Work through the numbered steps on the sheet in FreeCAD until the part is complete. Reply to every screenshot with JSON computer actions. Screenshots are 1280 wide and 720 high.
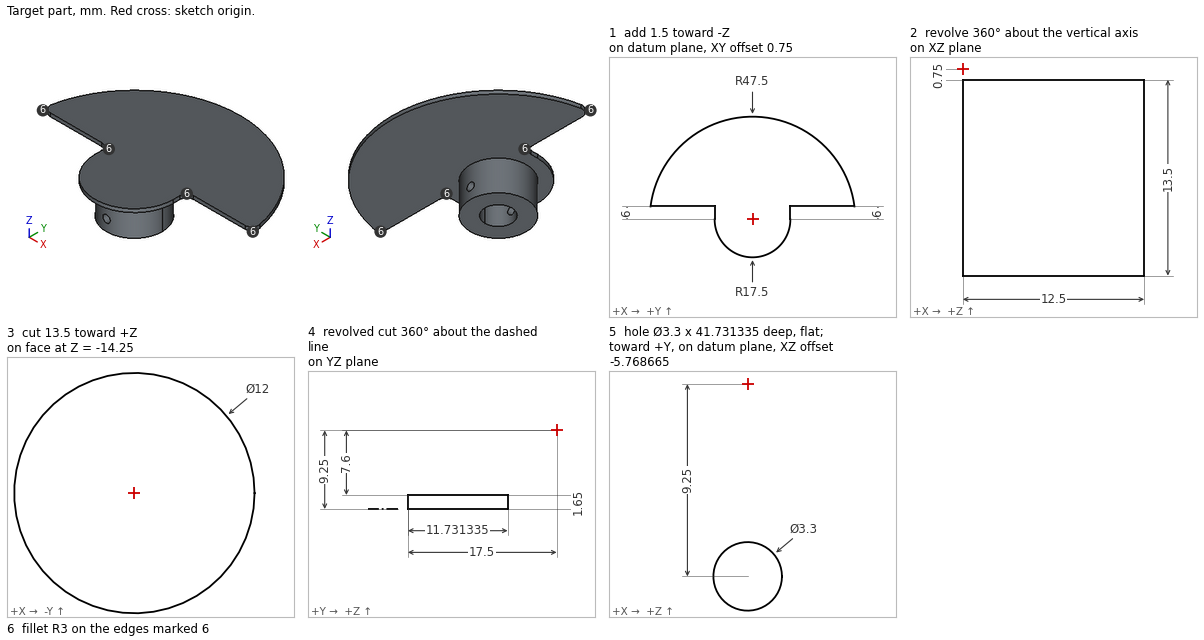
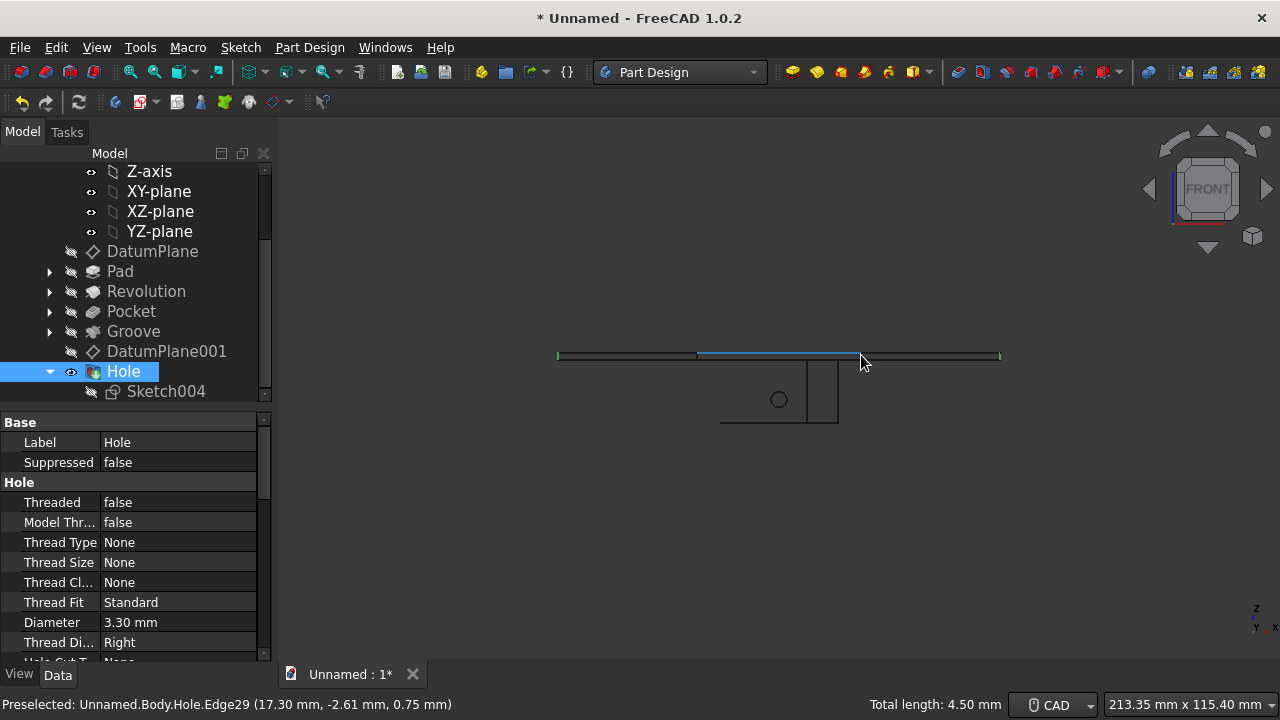
{"action": "key", "text": "3"}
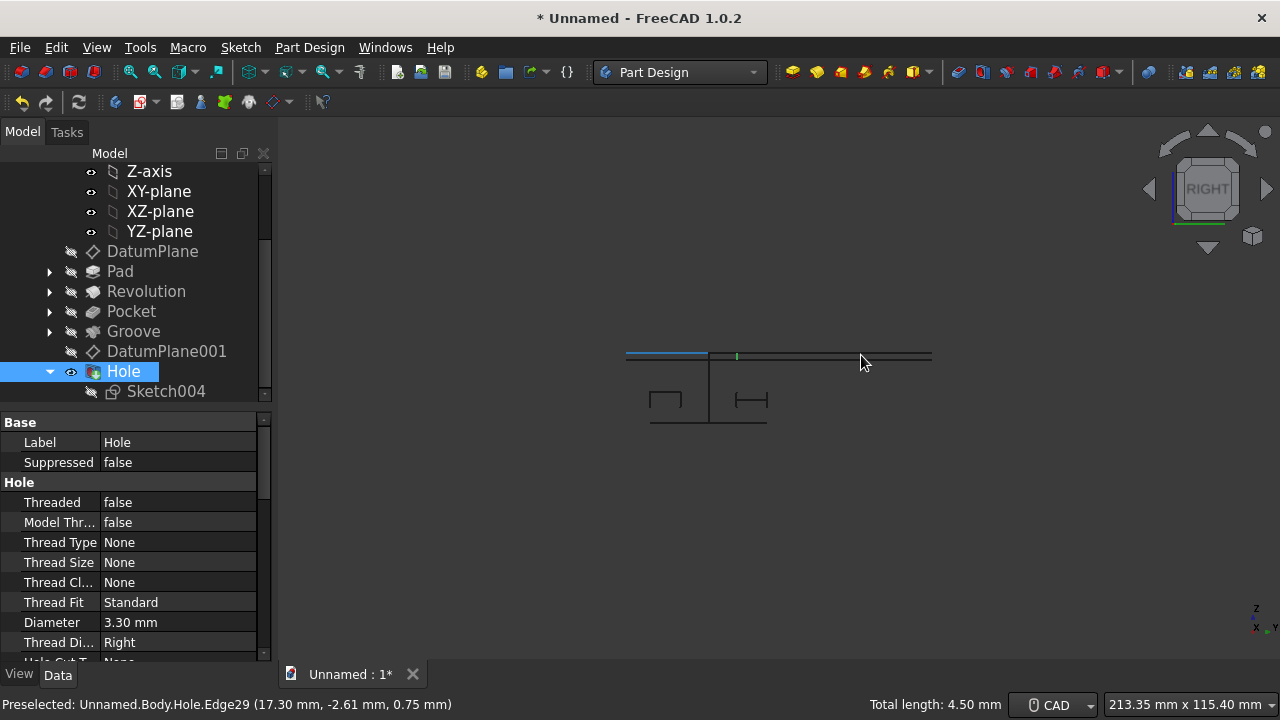
{"action": "left_click", "coordinate": [132, 72]}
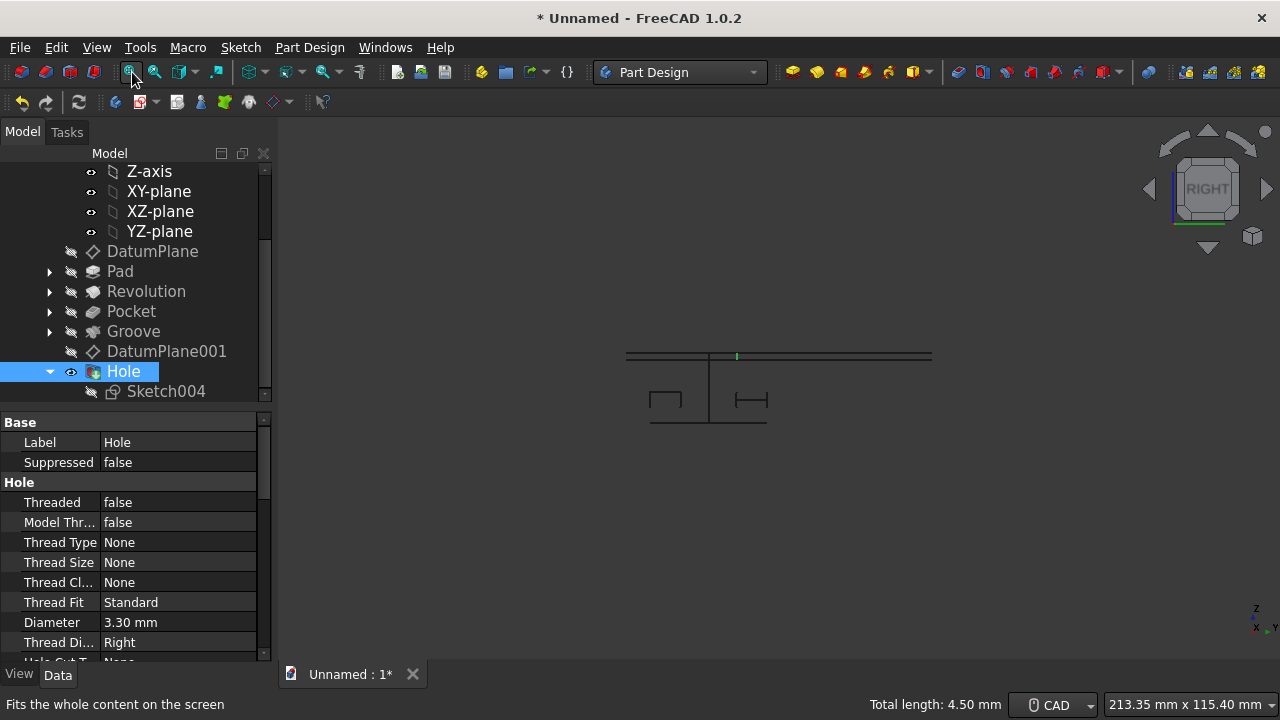
{"action": "scroll", "coordinate": [737, 355], "scroll_direction": "up", "scroll_amount": 9}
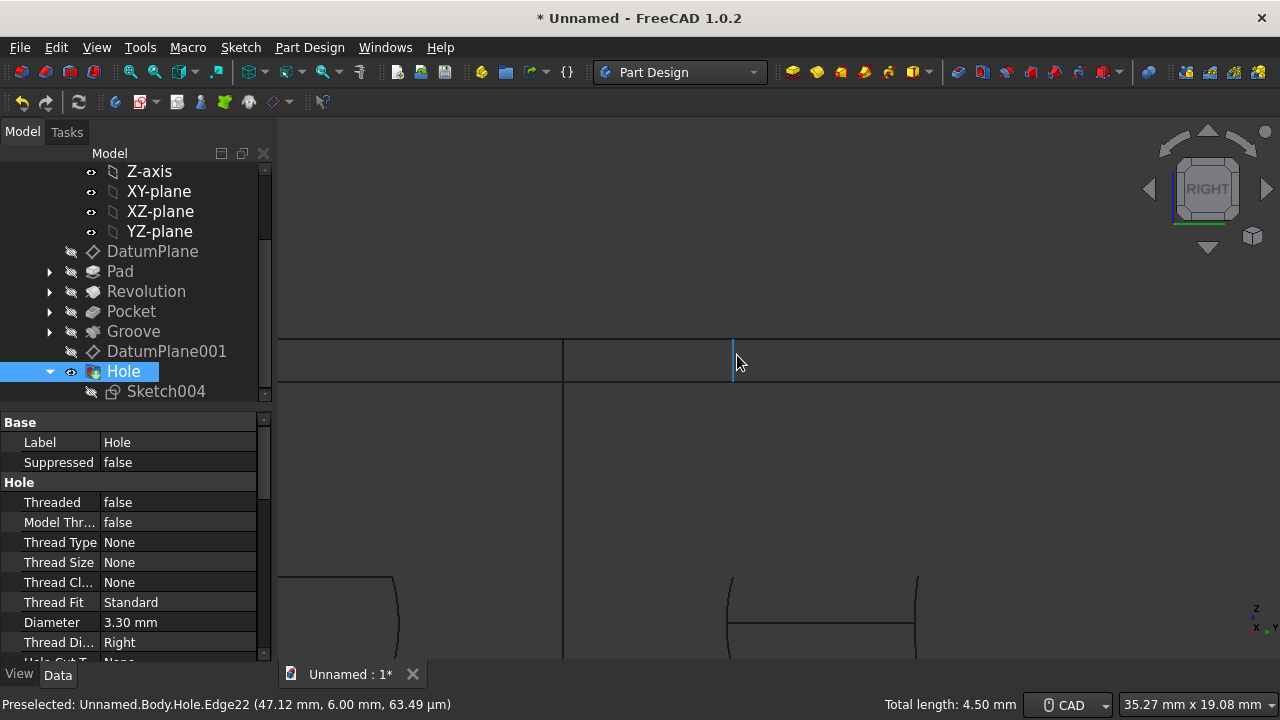
{"action": "key", "text": "v f"}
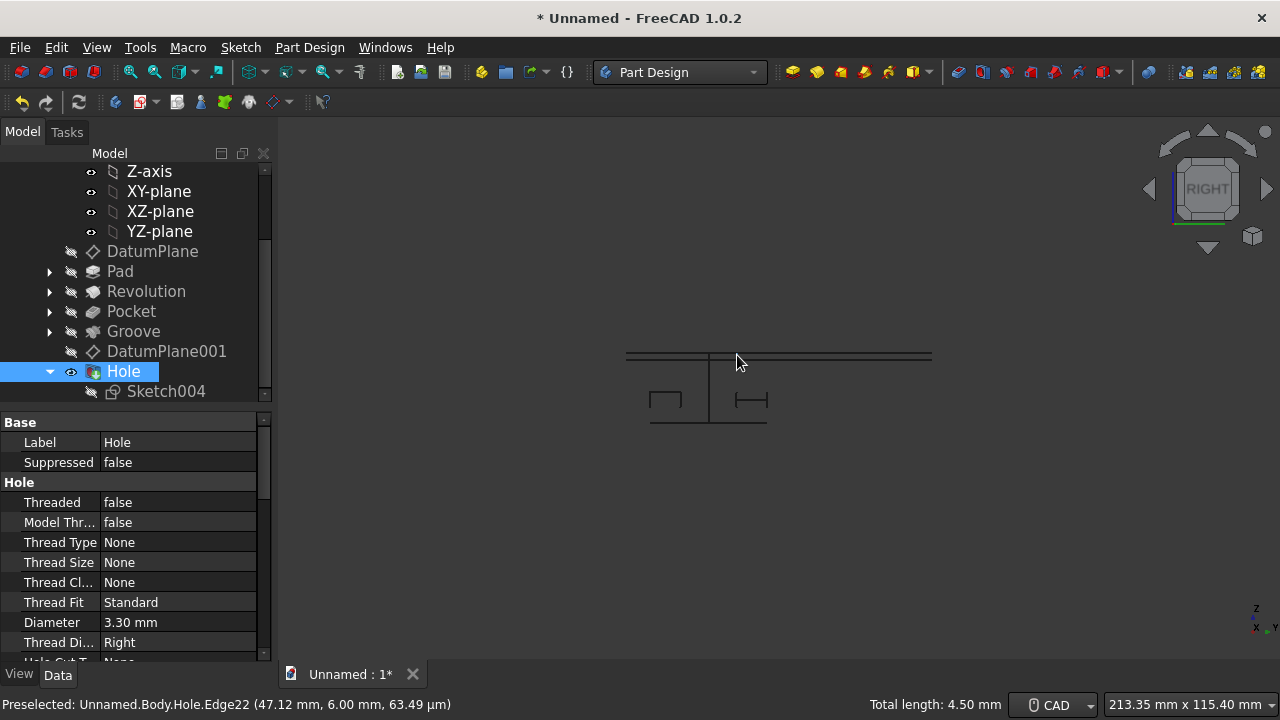
{"action": "key", "text": "5"}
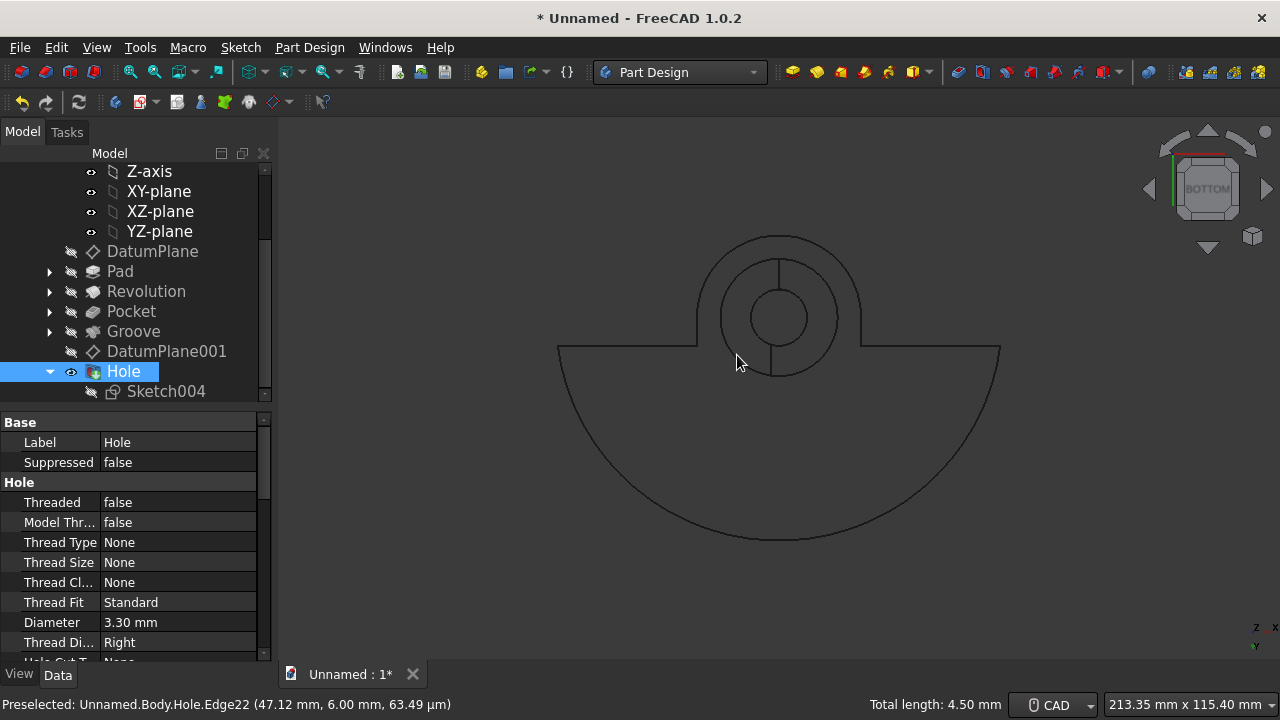
{"action": "scroll", "coordinate": [861, 345], "scroll_direction": "up", "scroll_amount": 9}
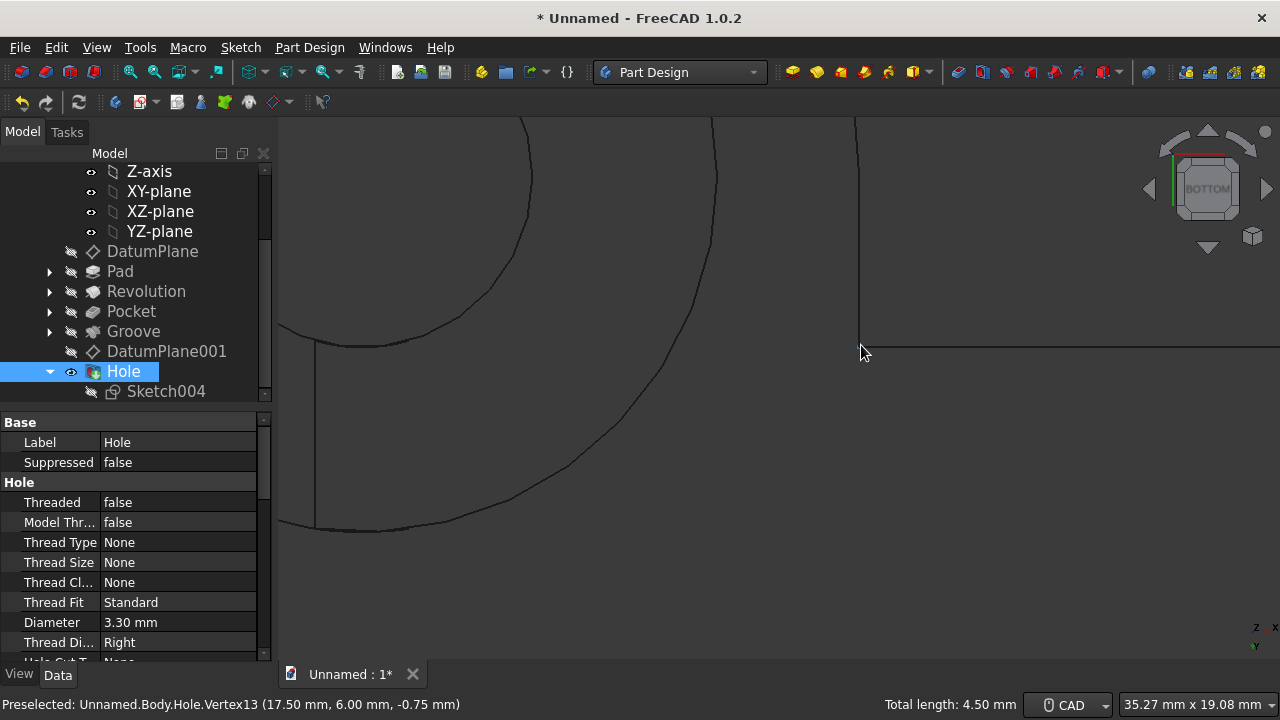
{"action": "key", "text": "v f"}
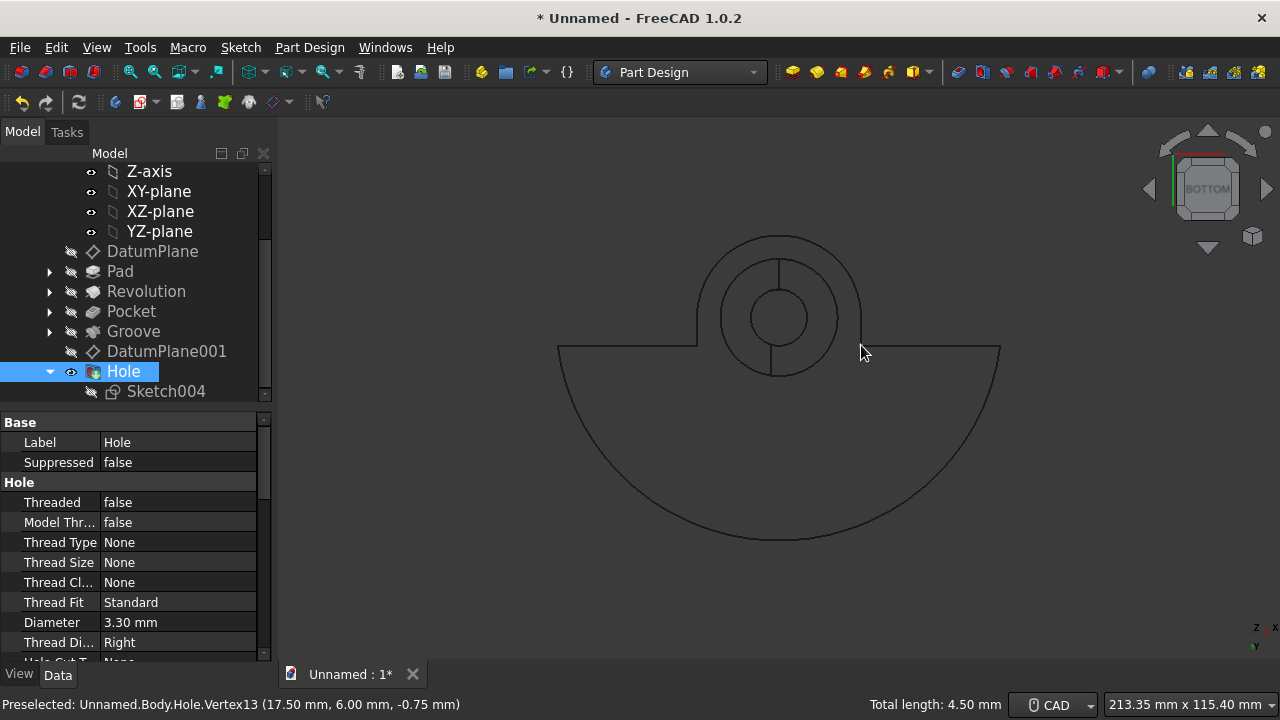
{"action": "key", "text": "4"}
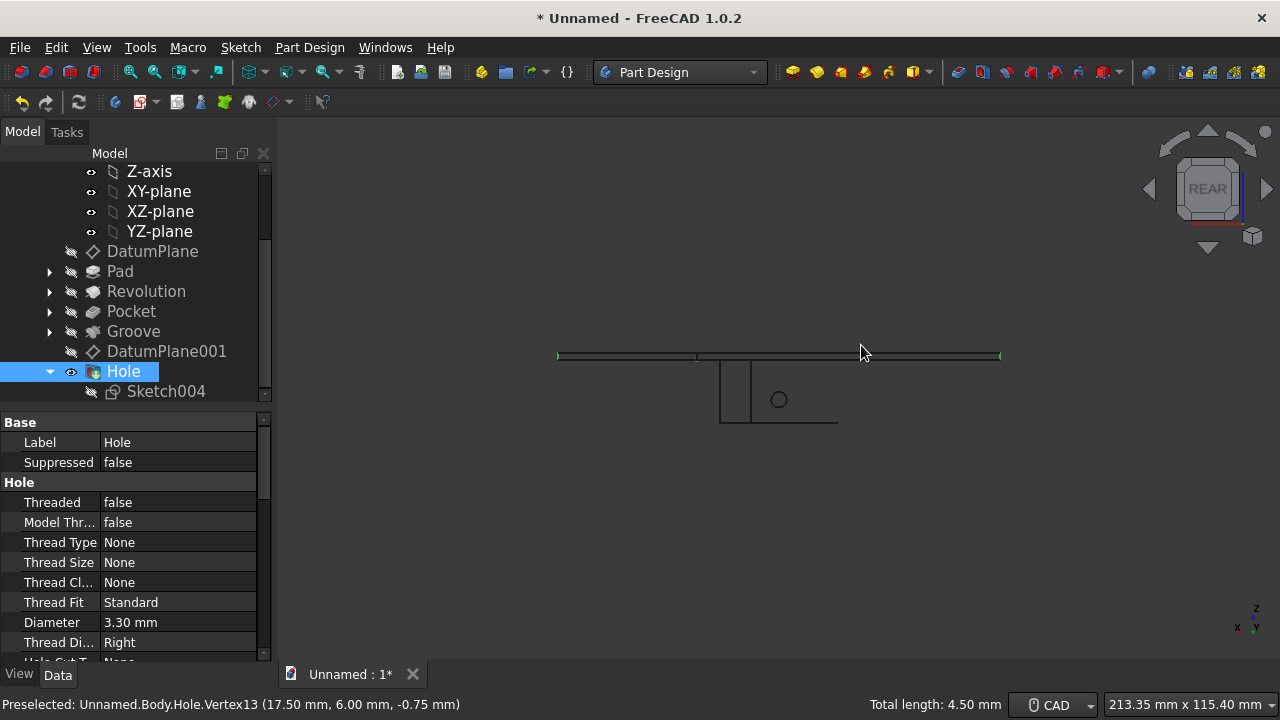
{"action": "key", "text": "v f"}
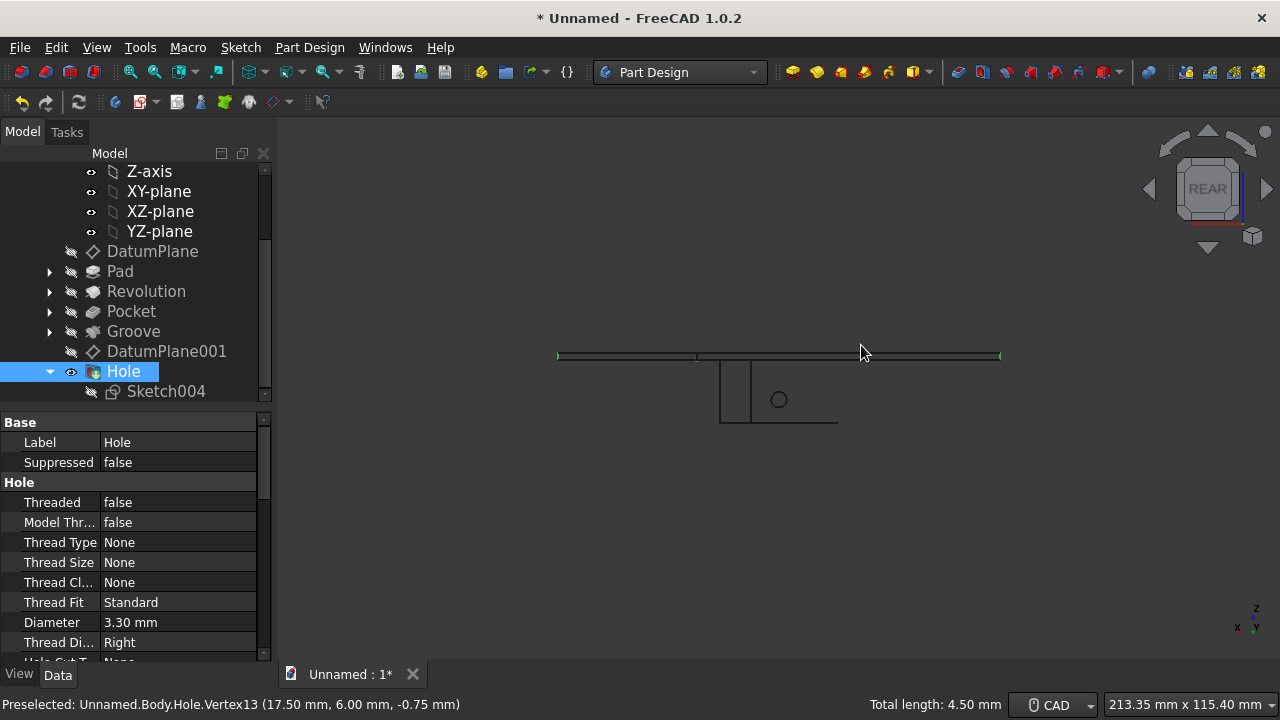
{"action": "scroll", "coordinate": [697, 355], "scroll_direction": "up", "scroll_amount": 9}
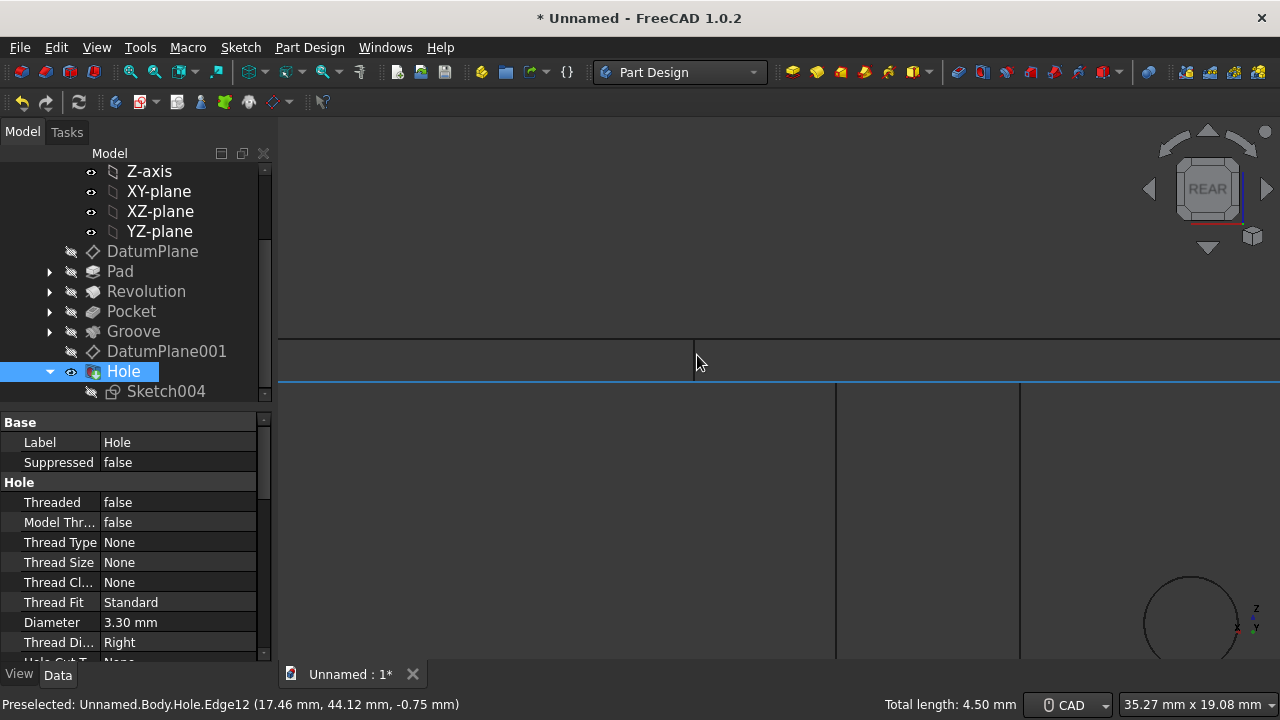
{"action": "left_click", "coordinate": [694, 360], "text": "ctrl"}